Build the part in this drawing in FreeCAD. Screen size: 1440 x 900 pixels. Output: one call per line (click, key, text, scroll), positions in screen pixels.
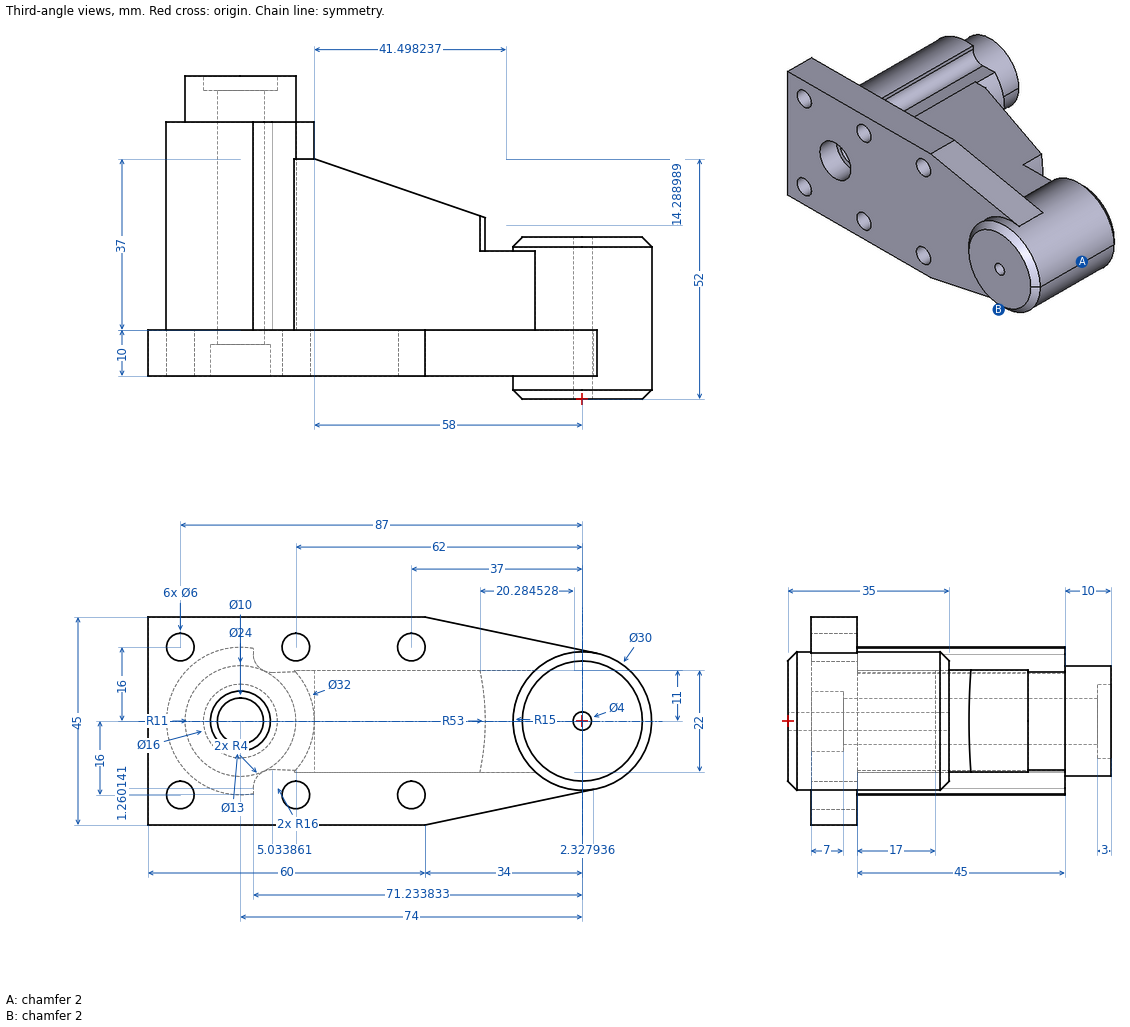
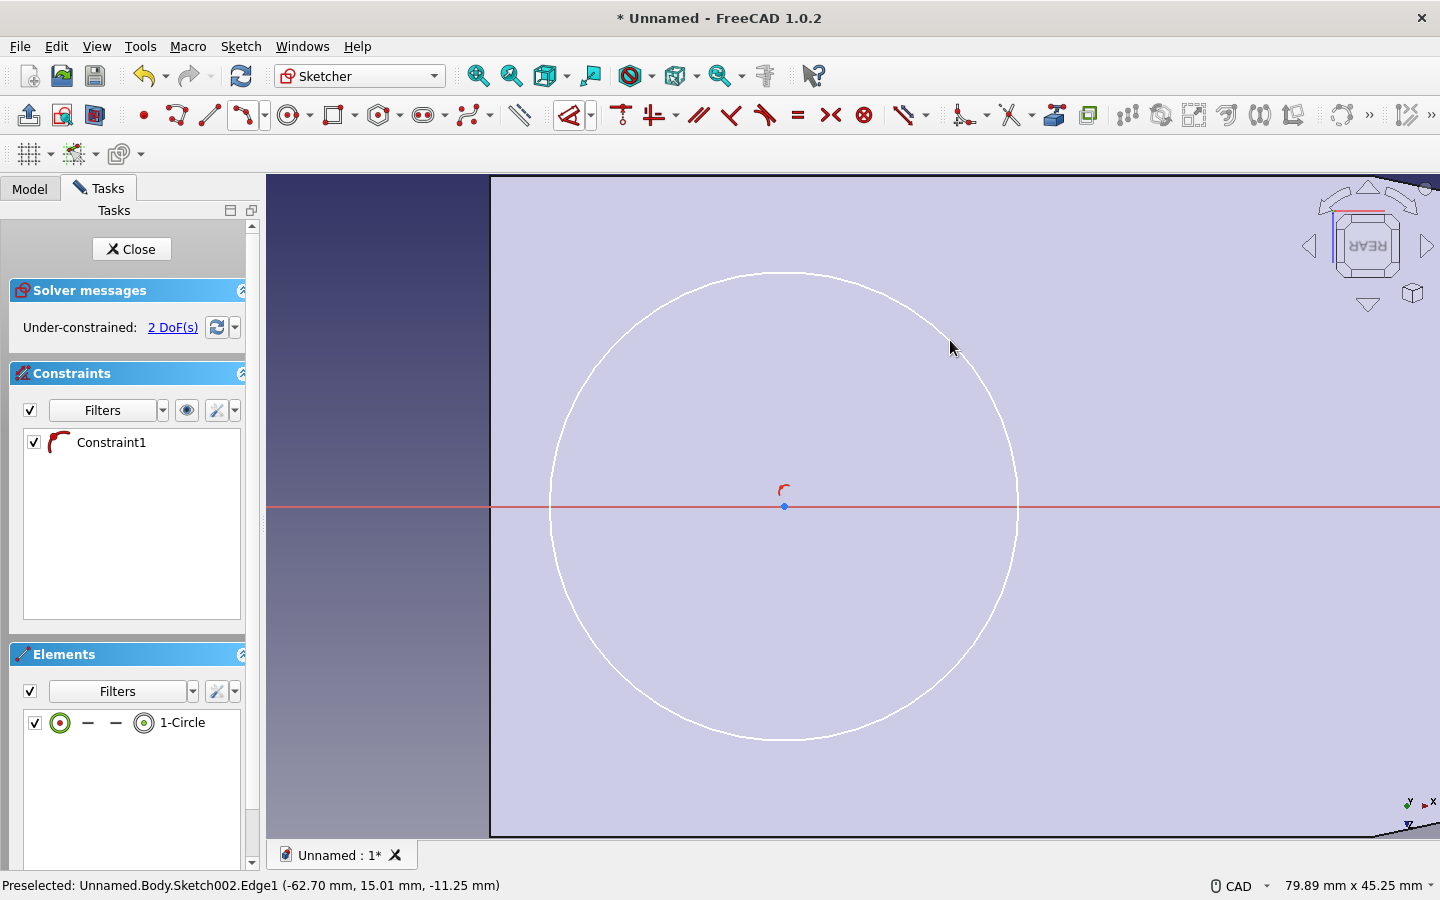
click(949, 340)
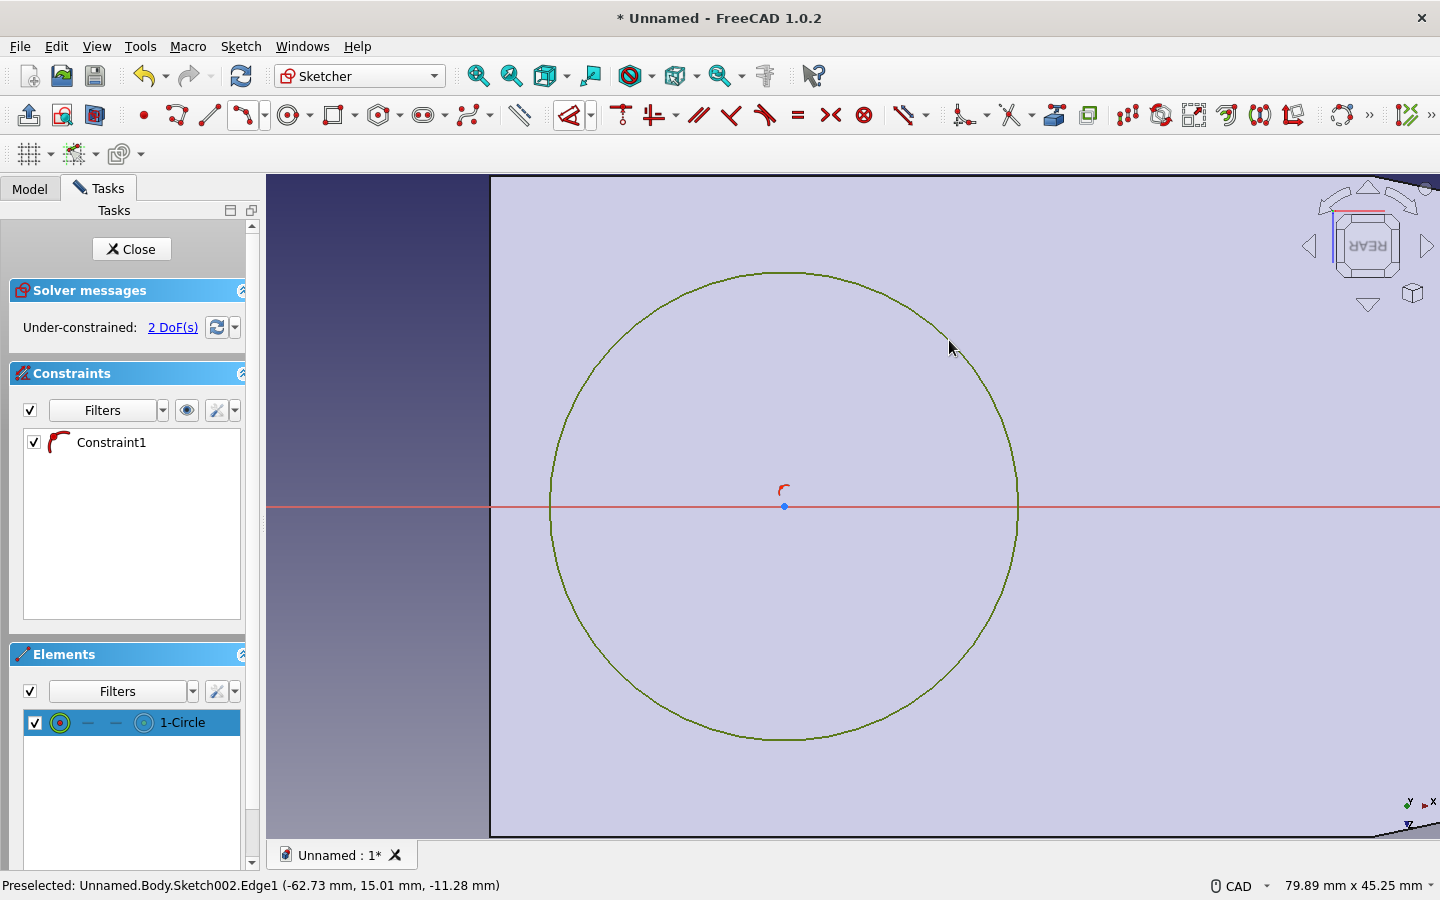
key(k)
key(o)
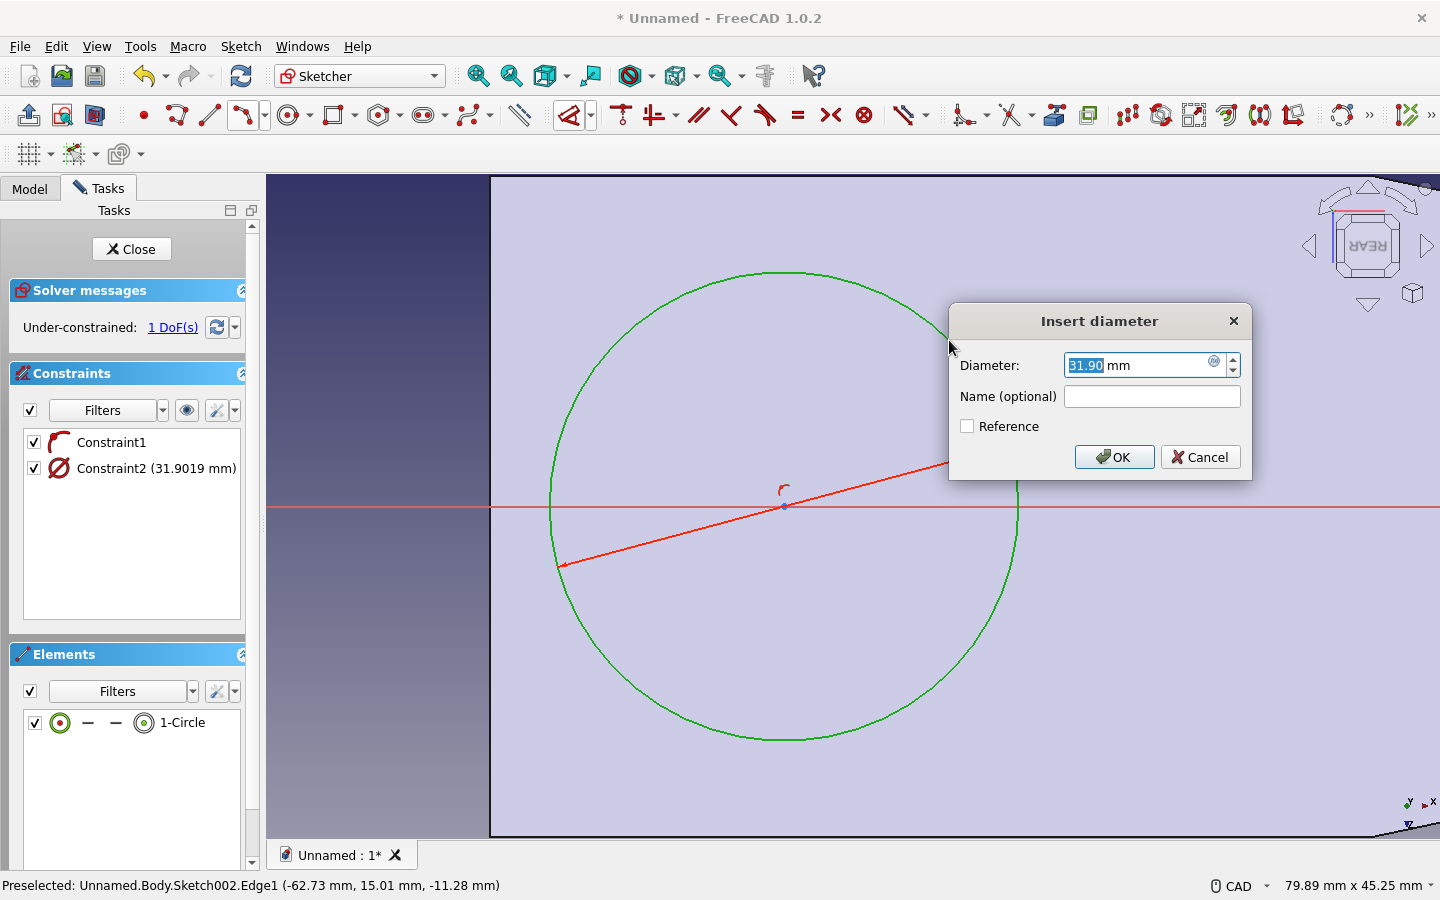
text(32)
key(Return)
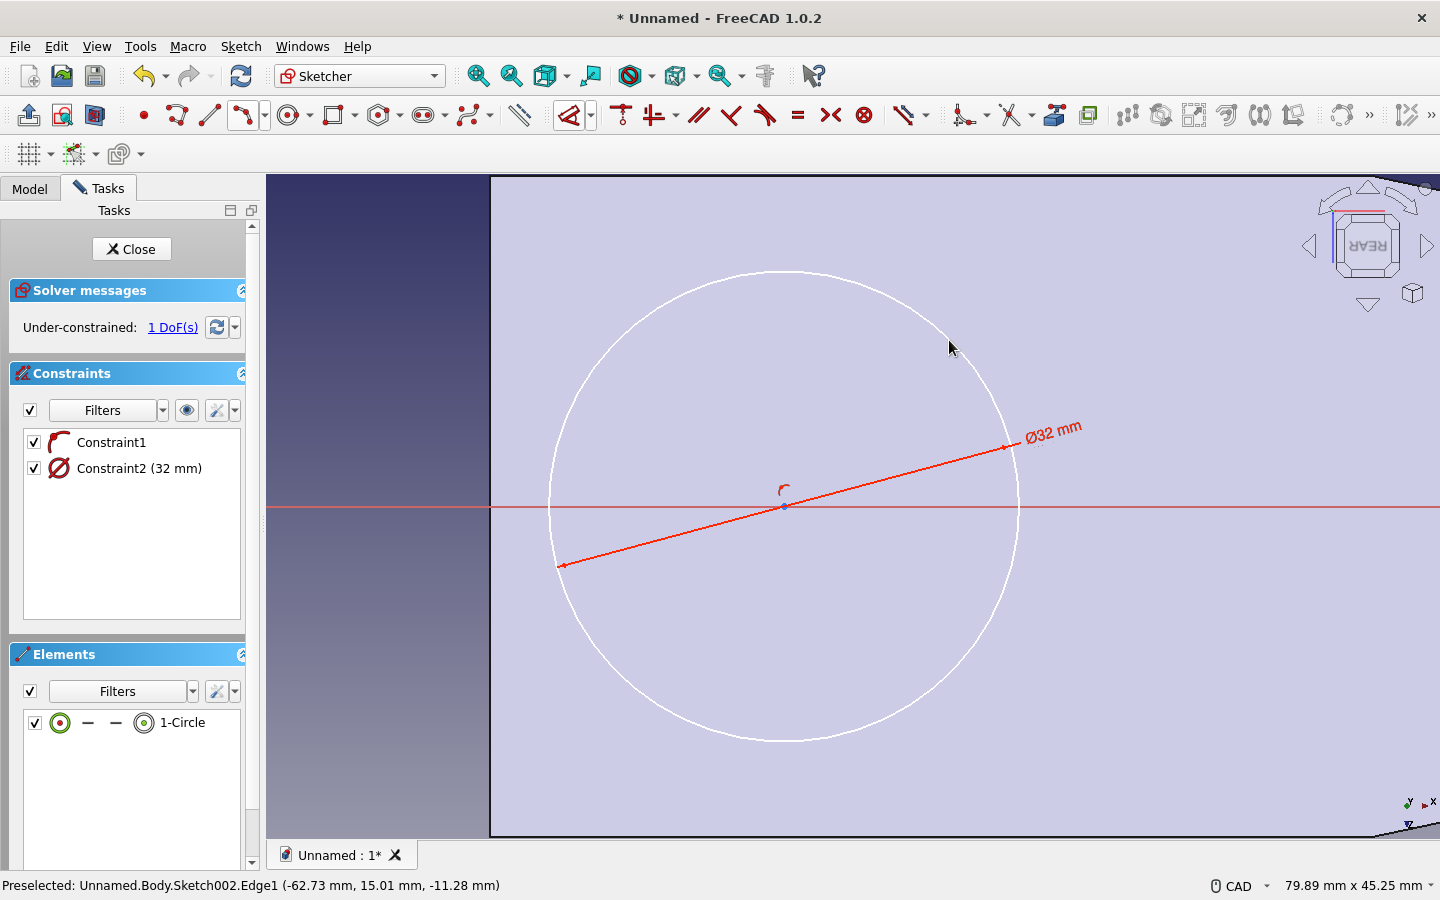
click(784, 506)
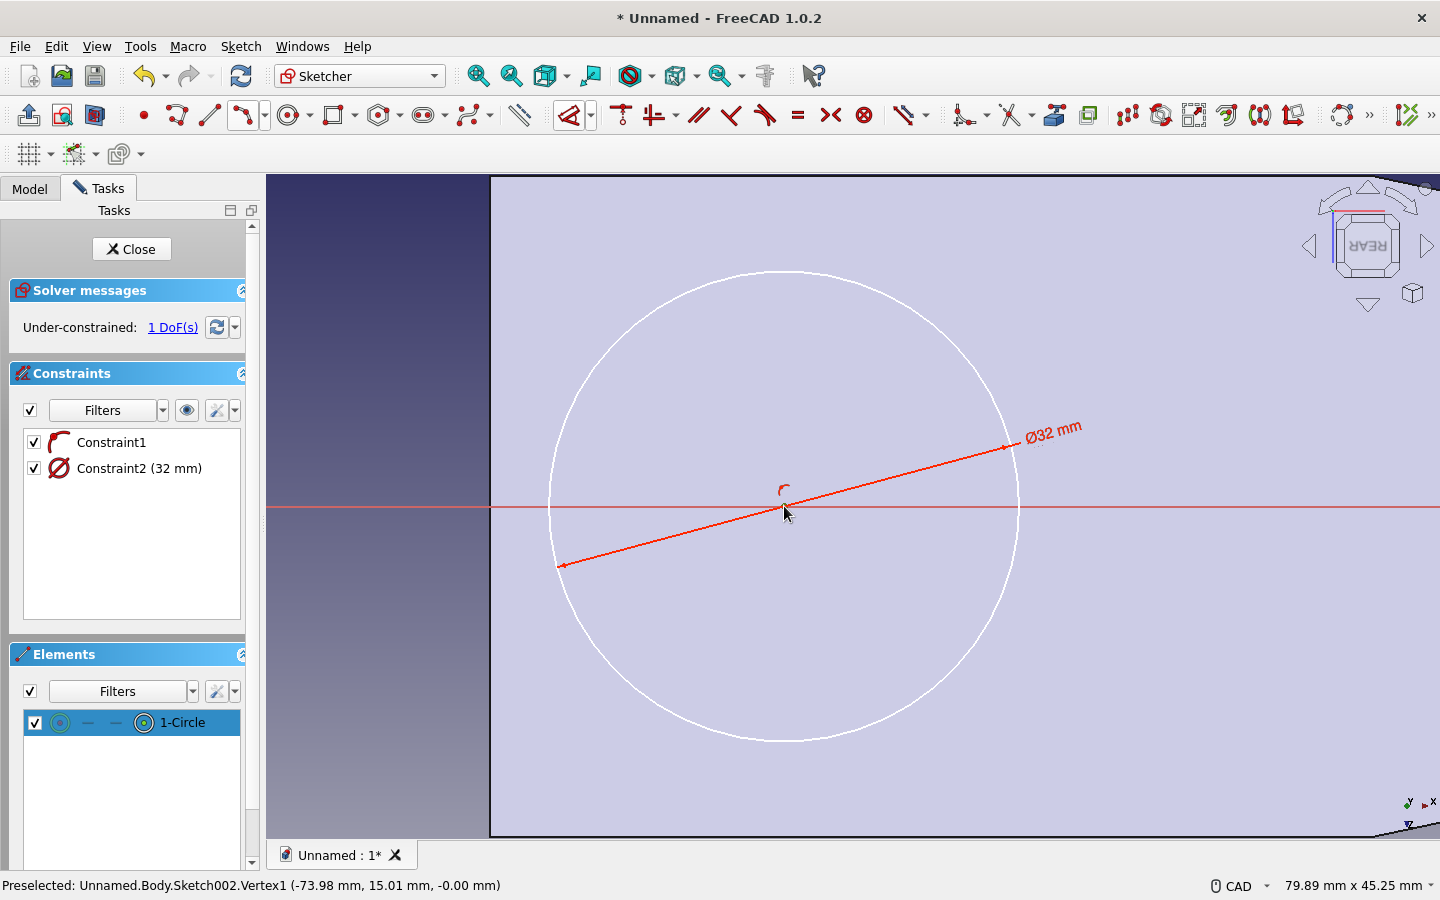
key(l)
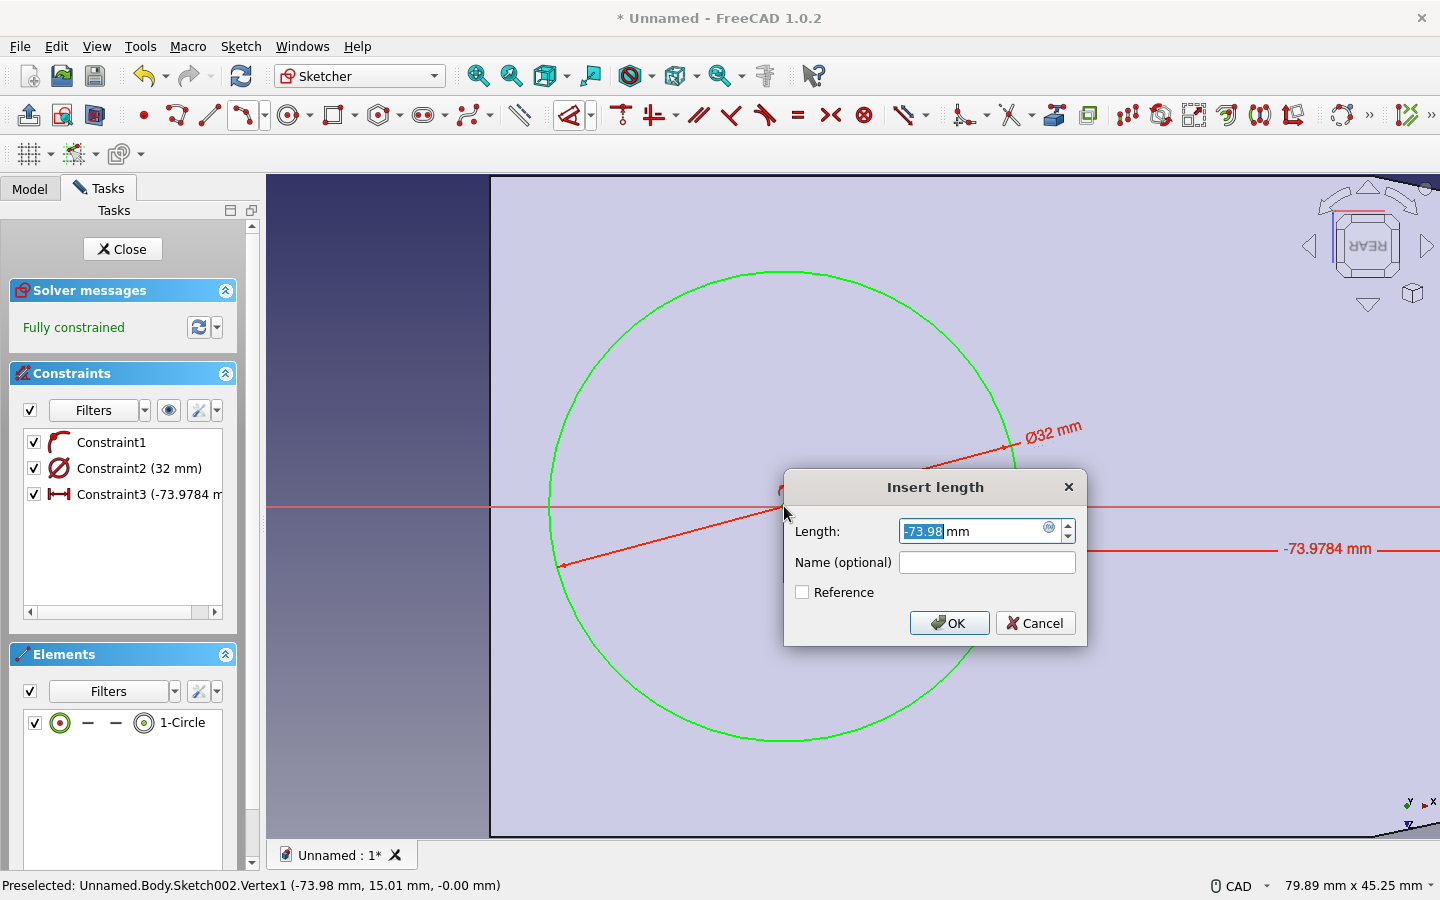
text(-74)
key(Return)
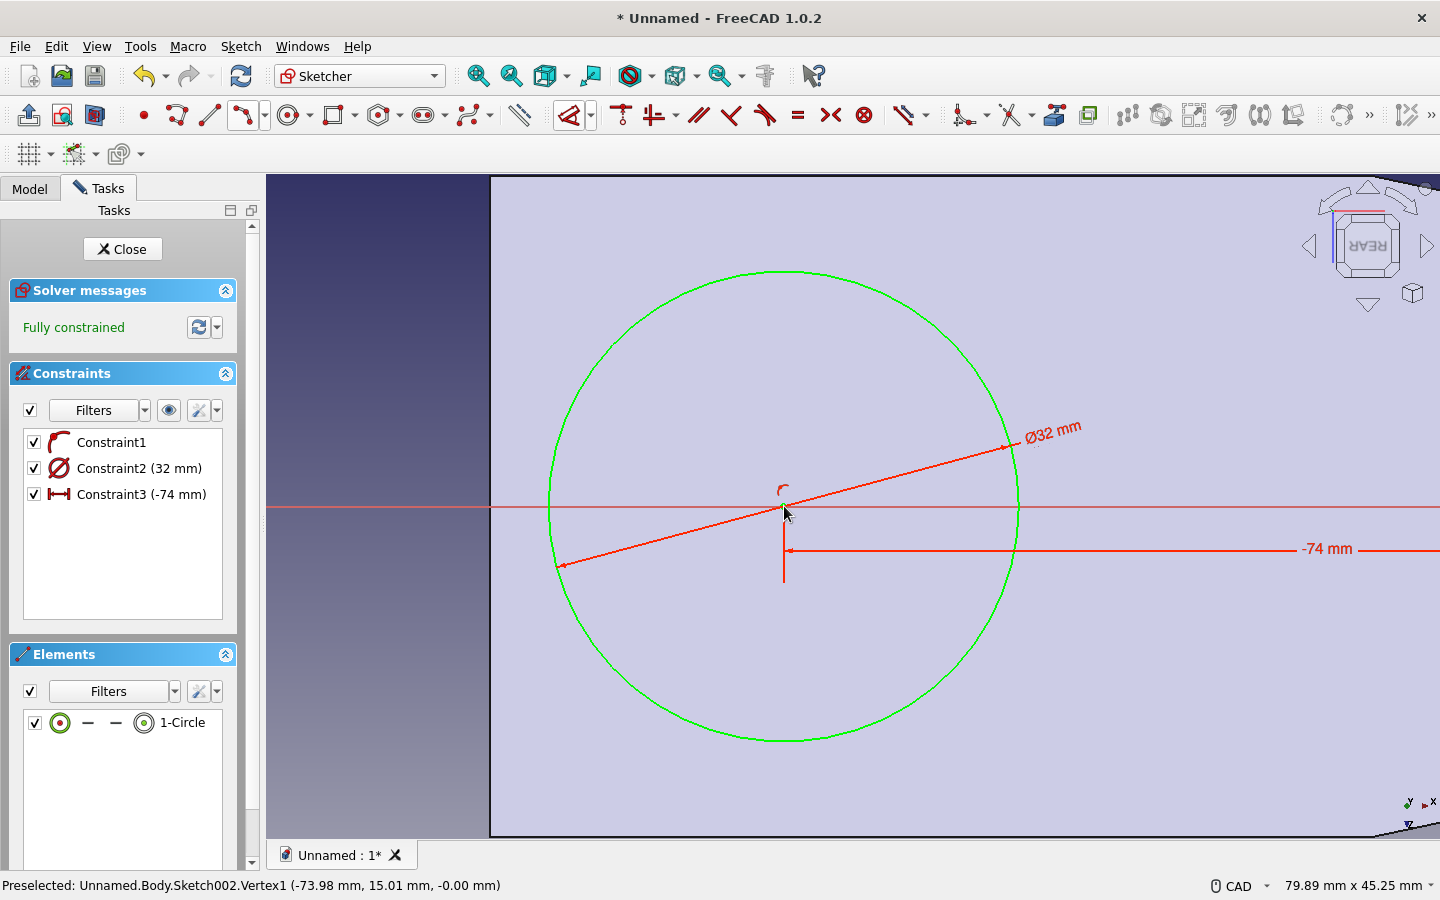
click(123, 249)